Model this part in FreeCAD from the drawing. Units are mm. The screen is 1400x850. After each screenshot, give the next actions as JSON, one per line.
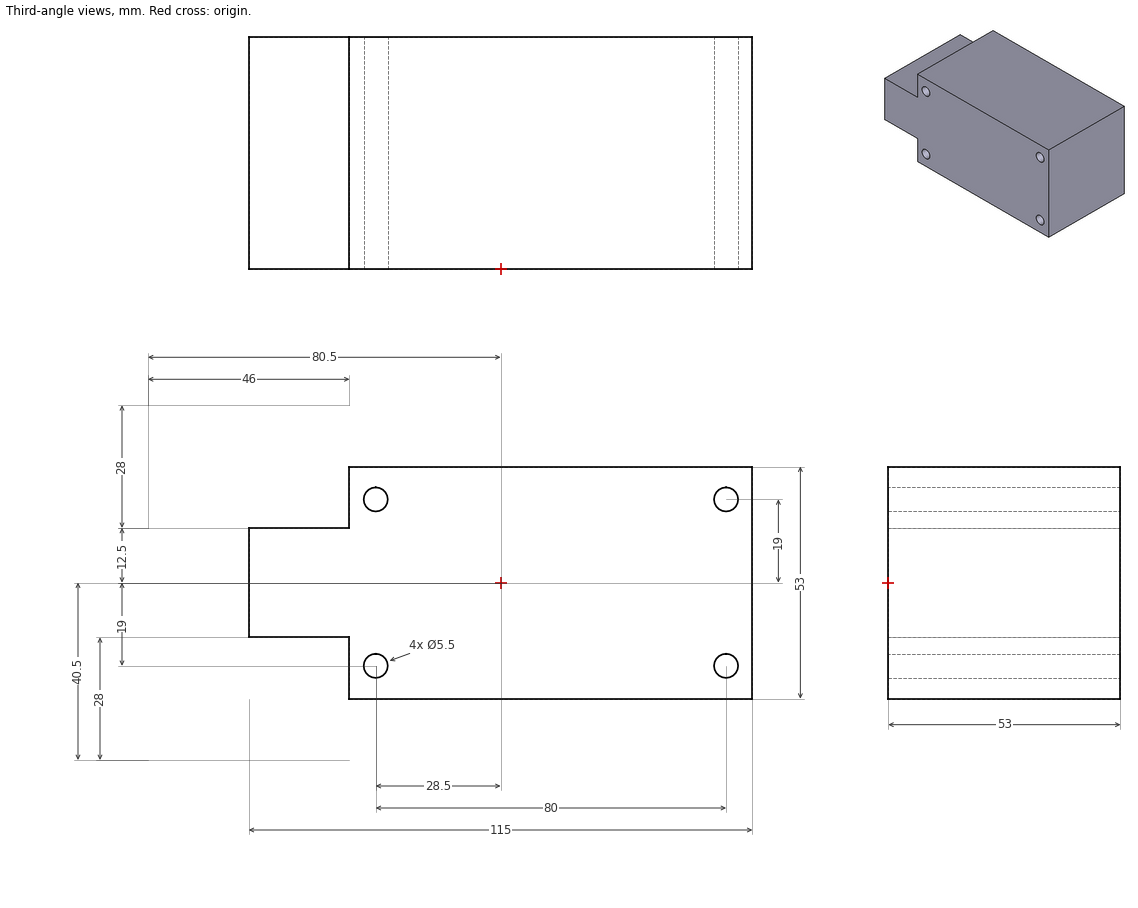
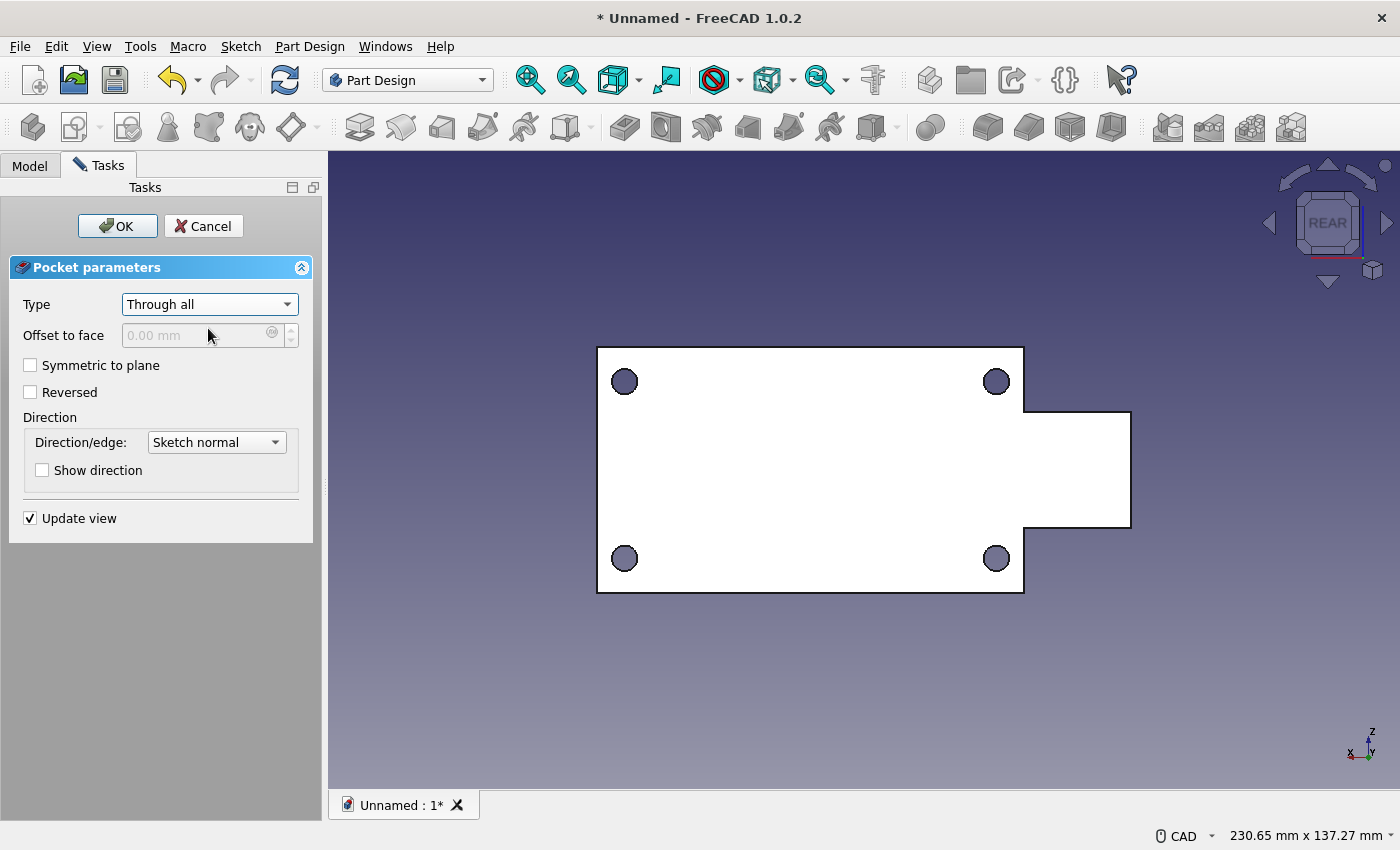
{"action": "left_click", "coordinate": [118, 226]}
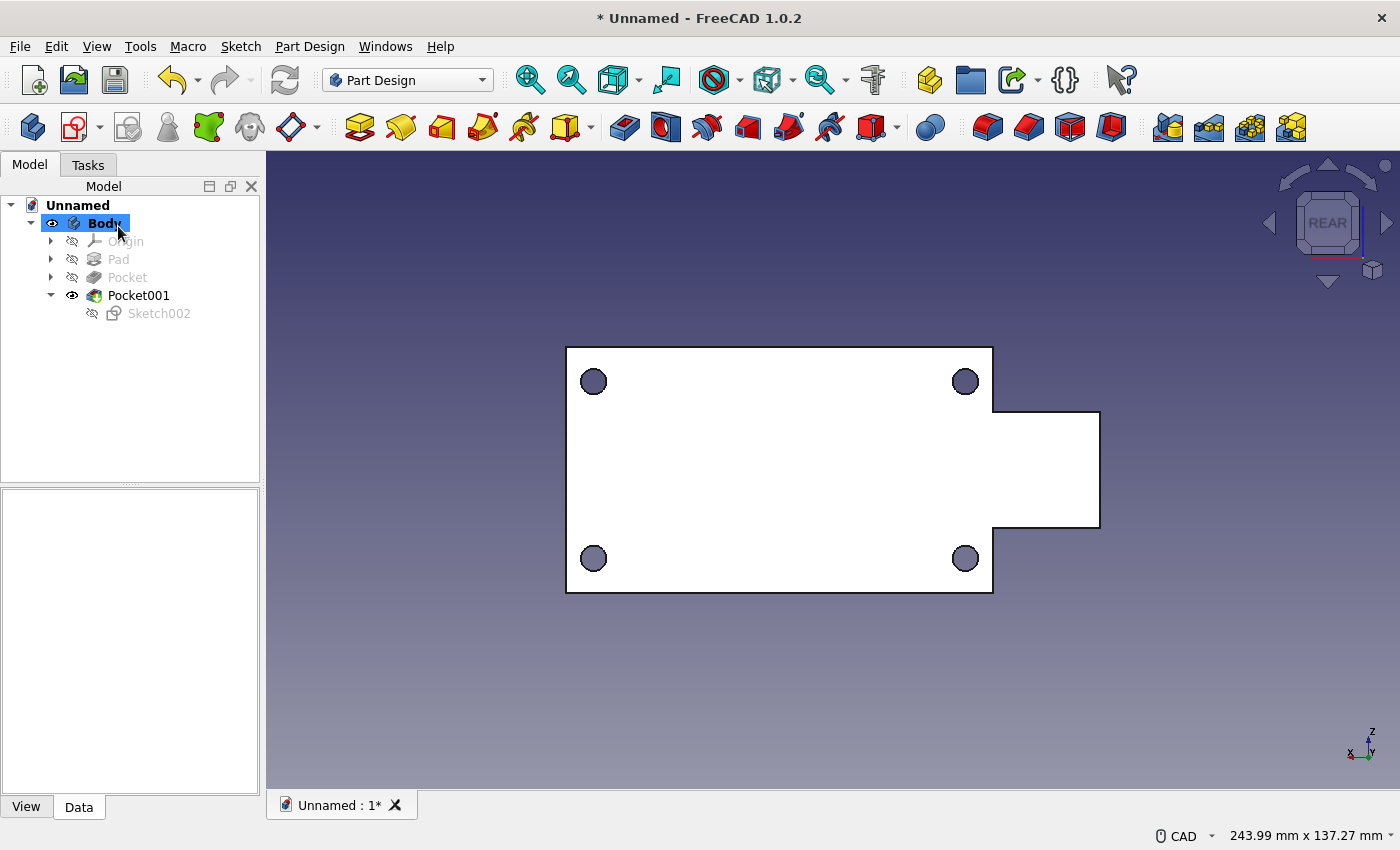
{"action": "key", "text": "0"}